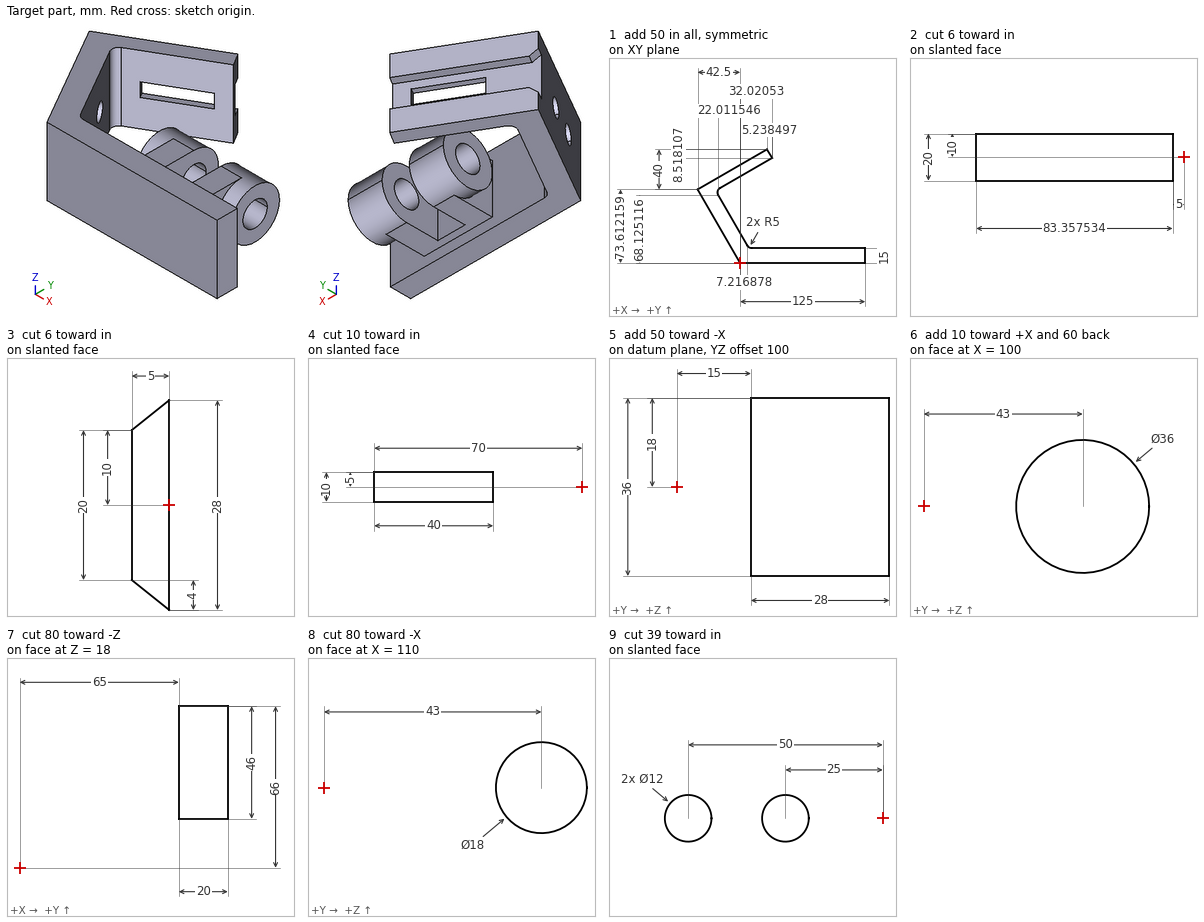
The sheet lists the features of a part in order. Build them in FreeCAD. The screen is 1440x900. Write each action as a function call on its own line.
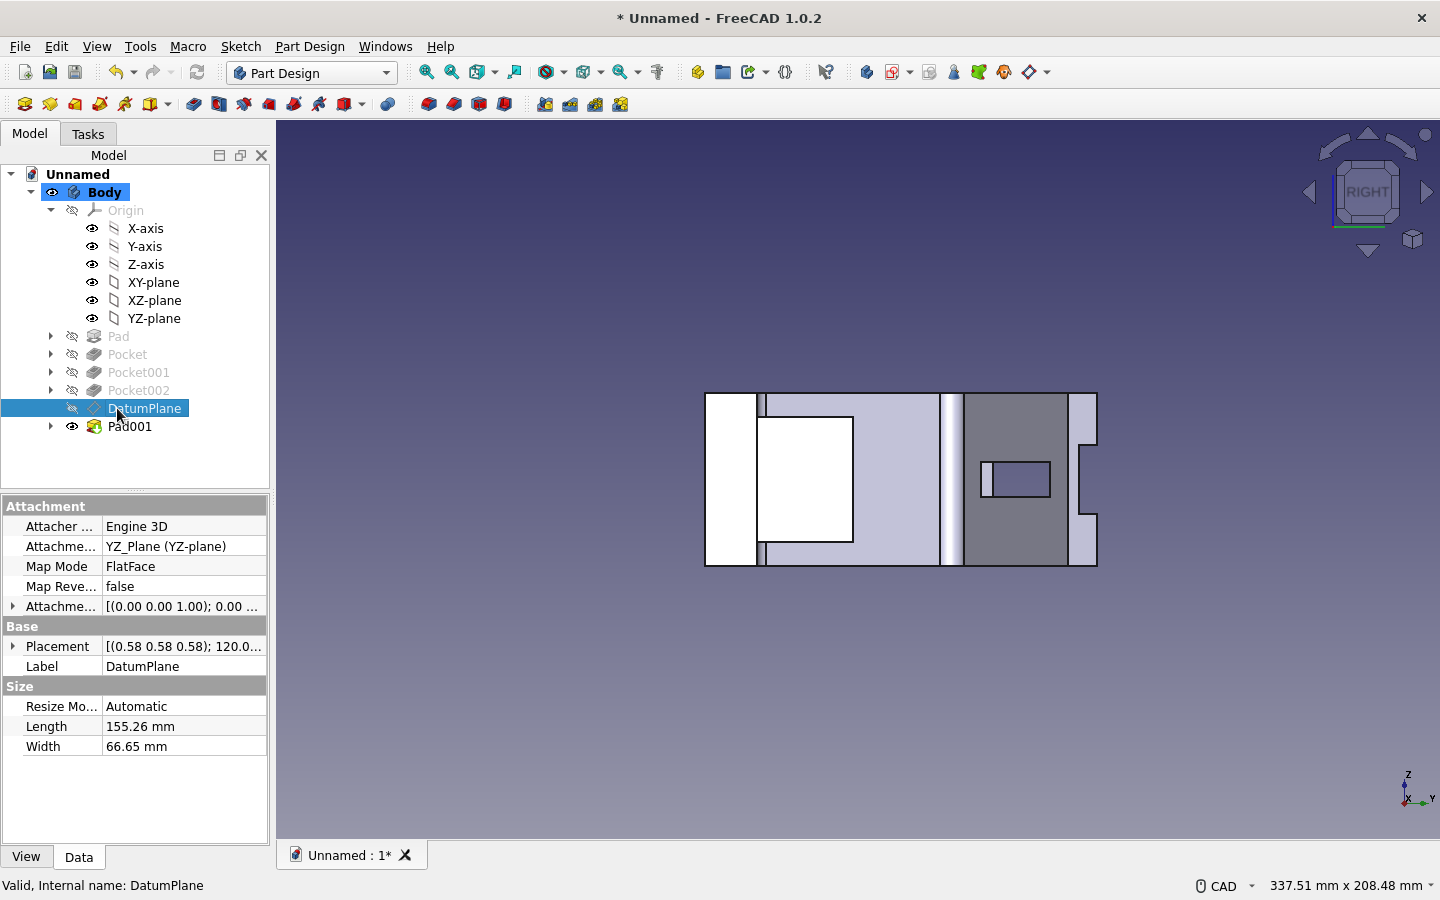
click(427, 72)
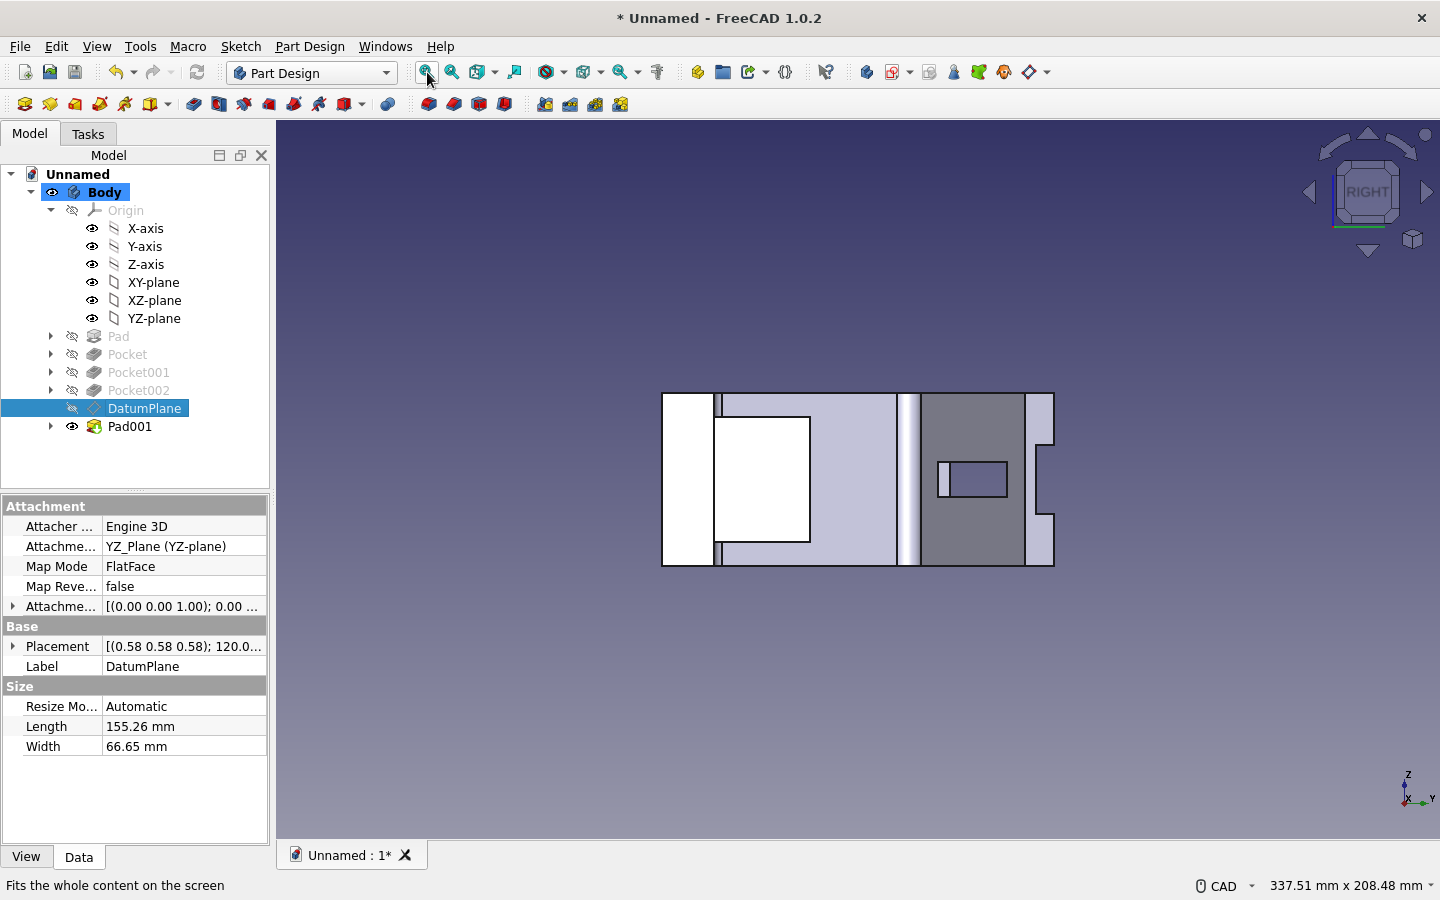
click(762, 478)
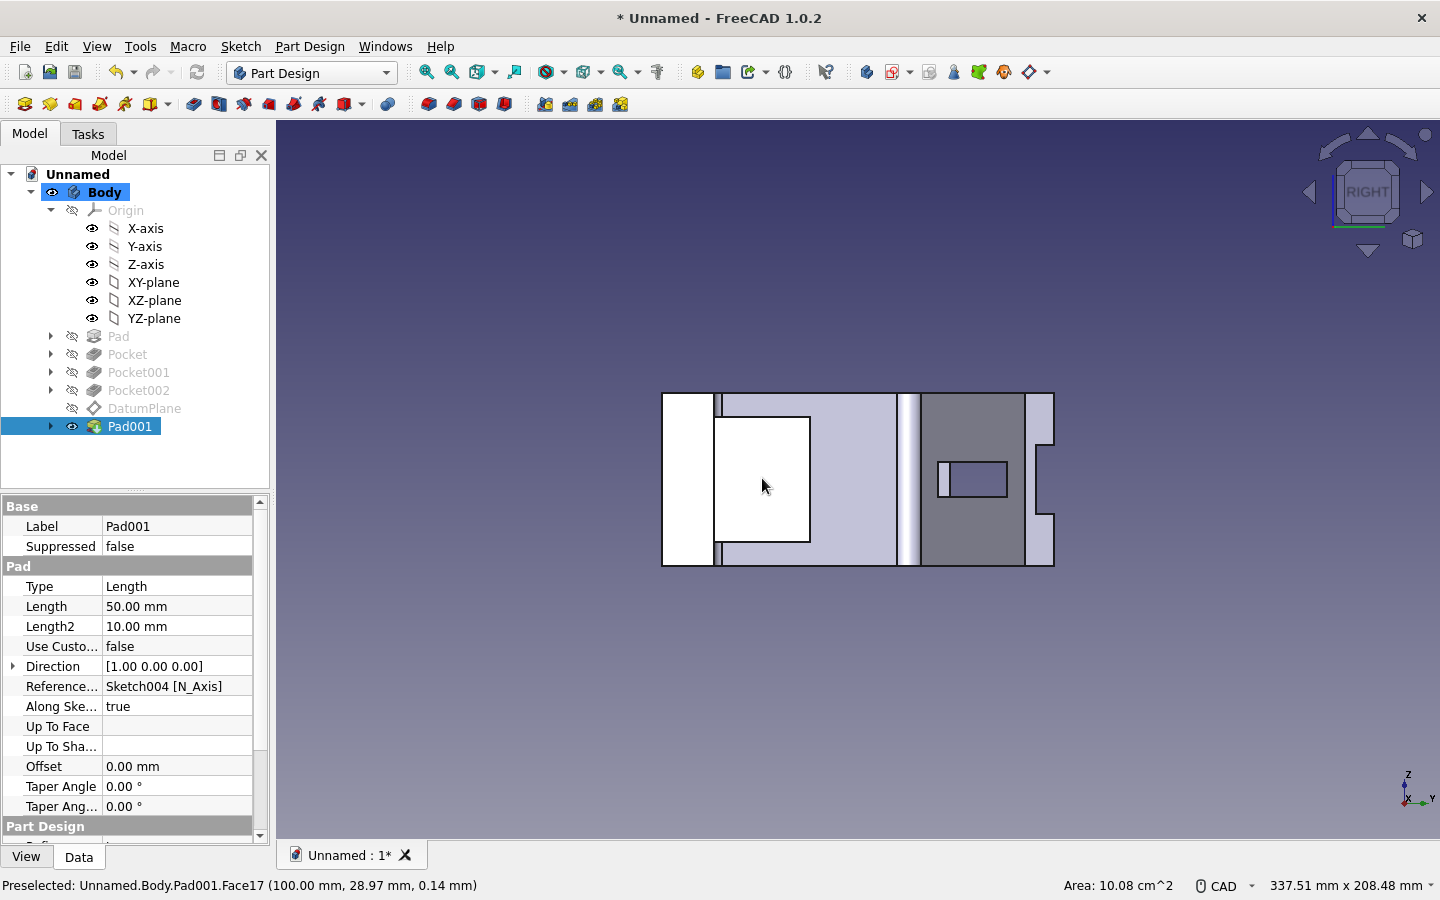
click(892, 72)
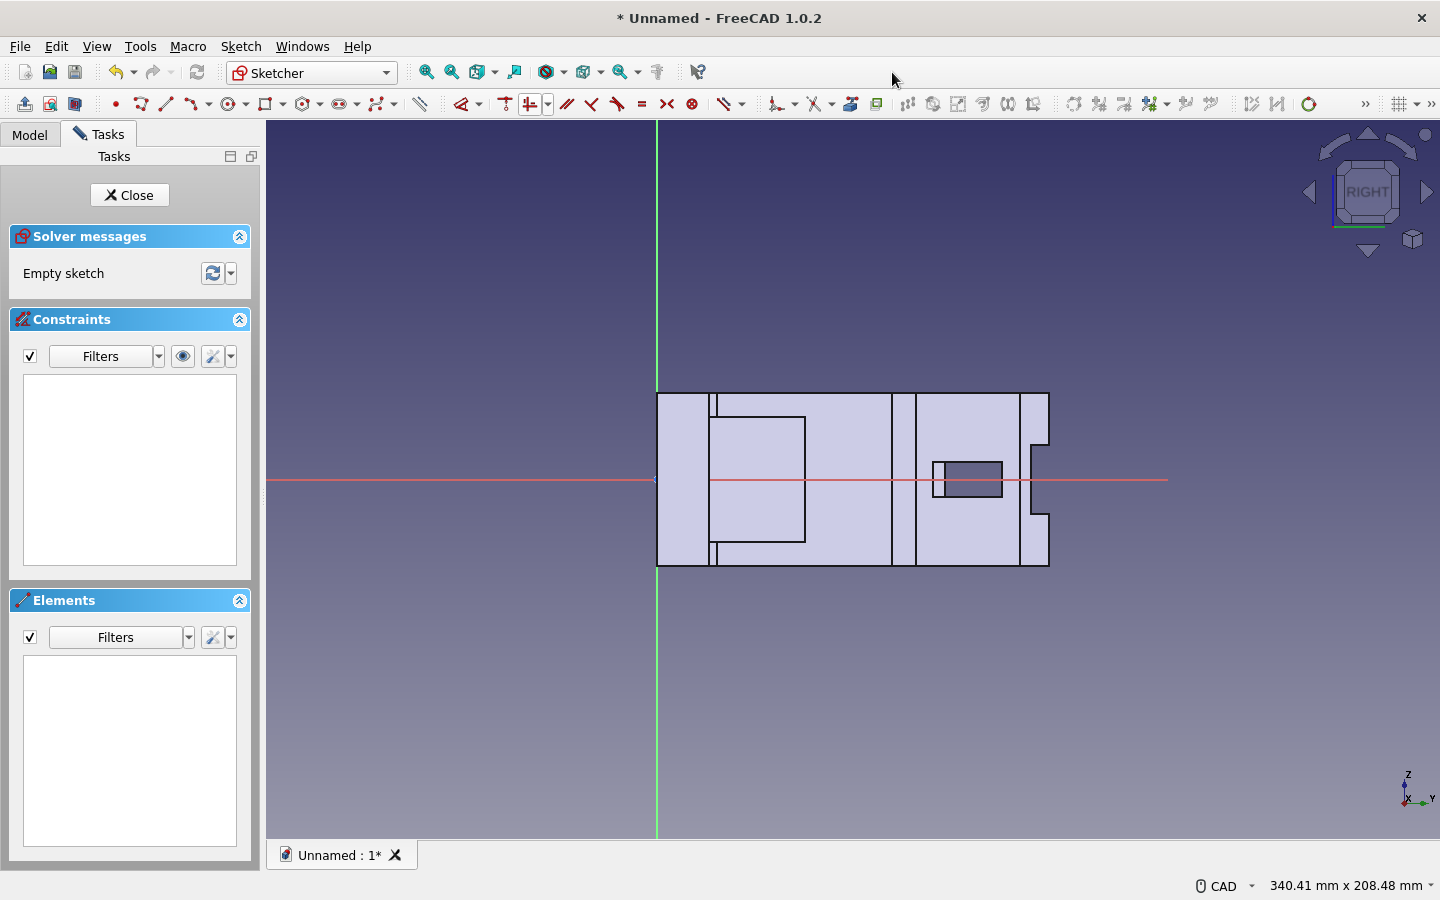
scroll(753, 480, up, 6)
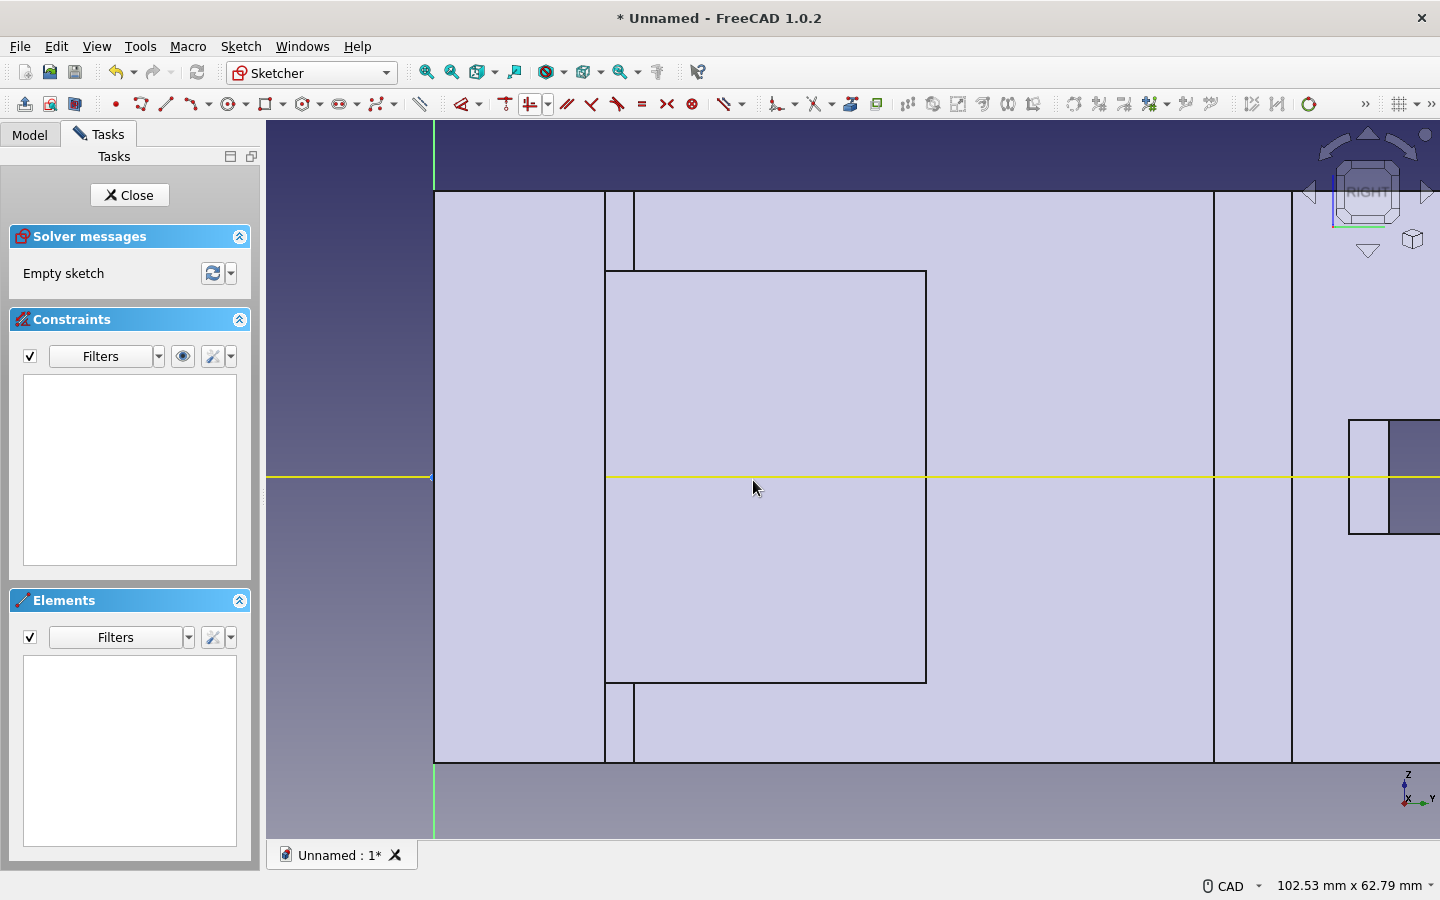
click(228, 104)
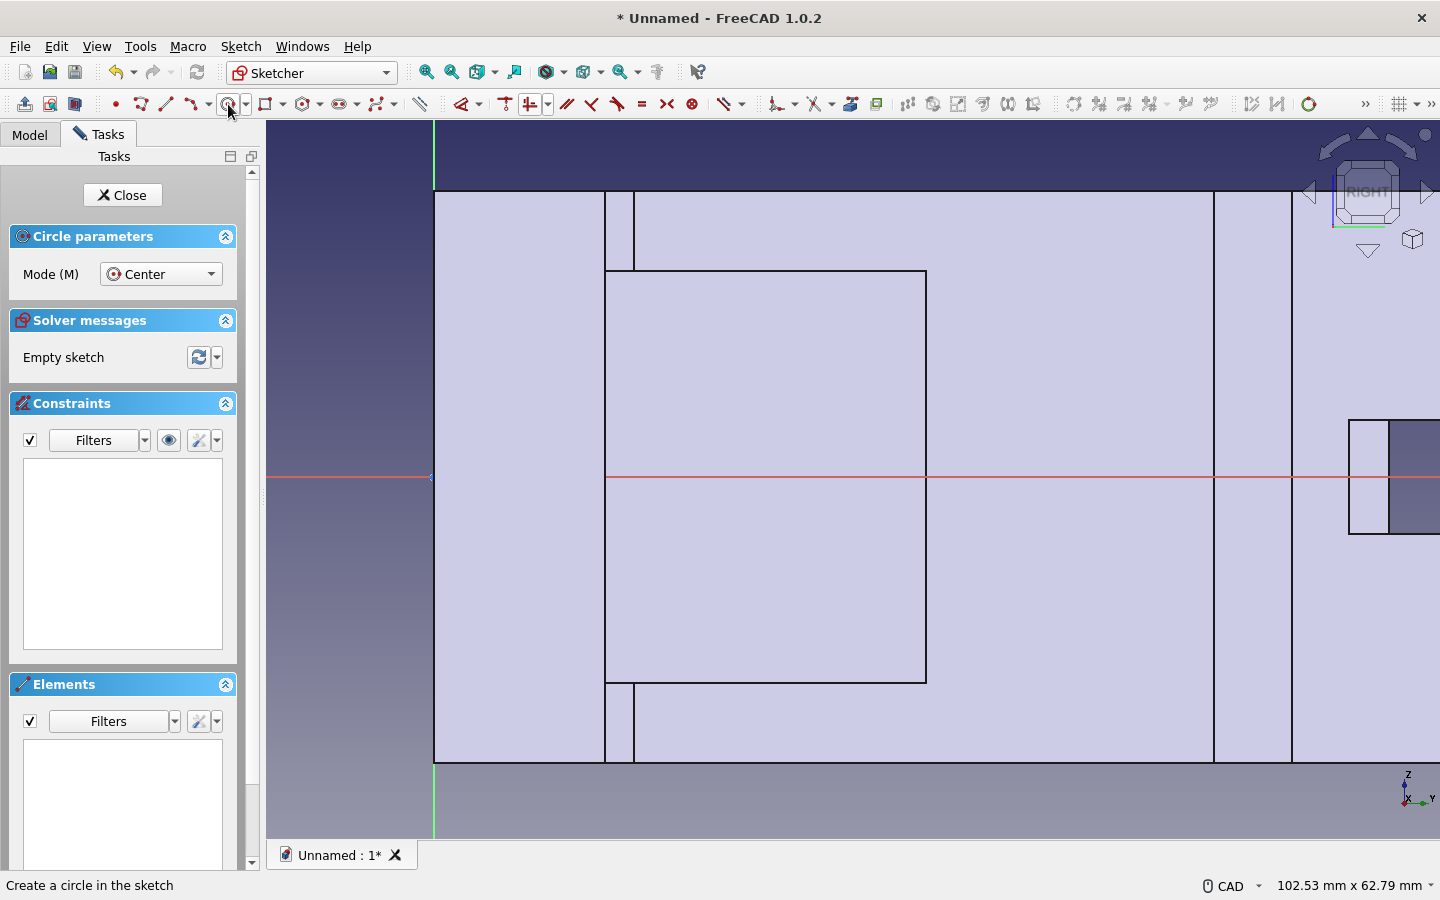
click(926, 477)
click(1072, 331)
key(Escape)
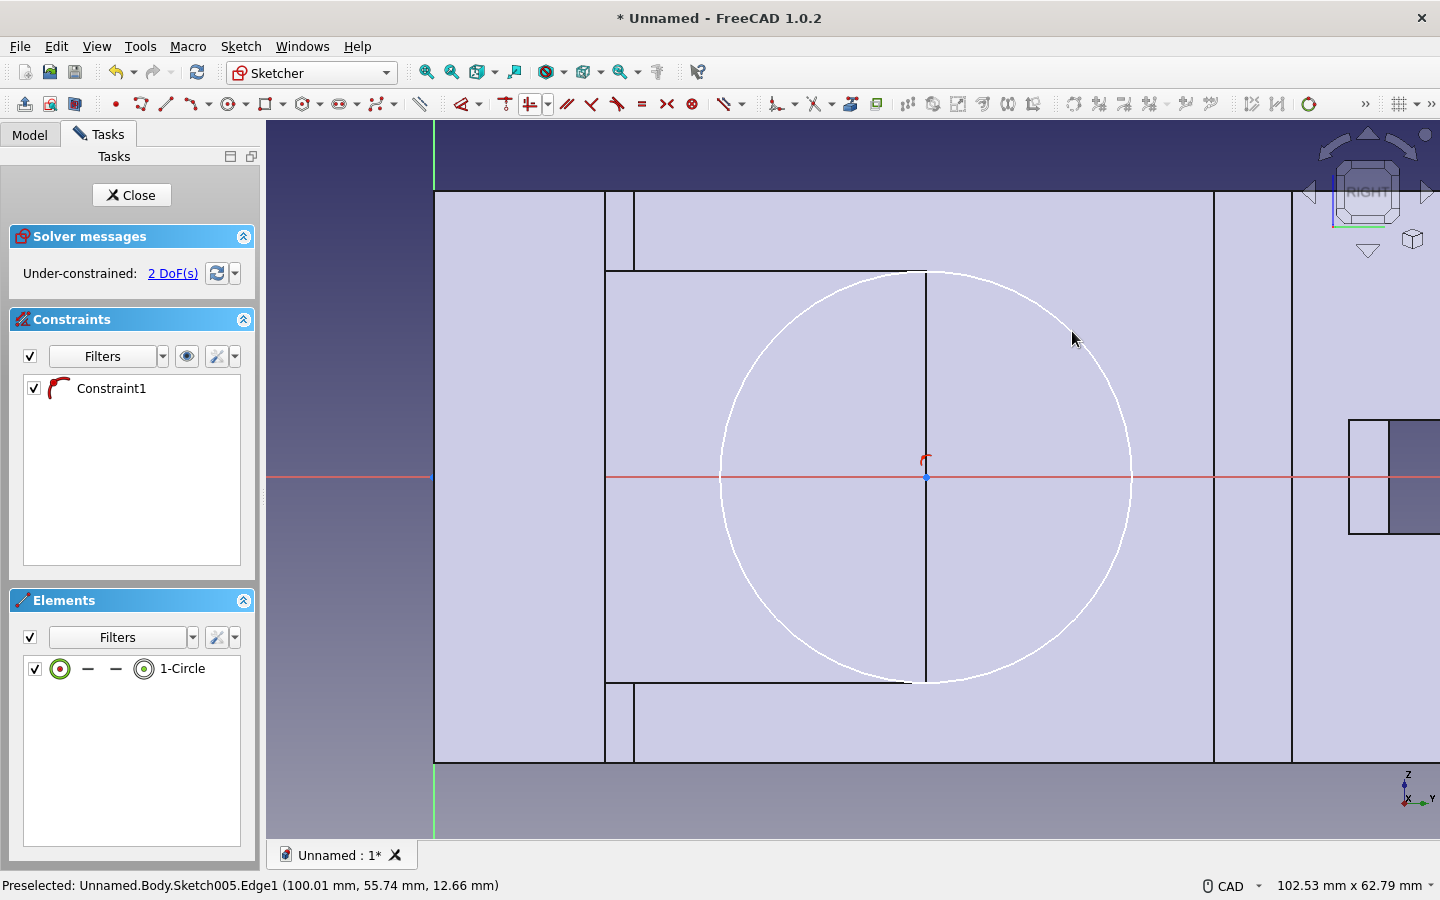
click(460, 104)